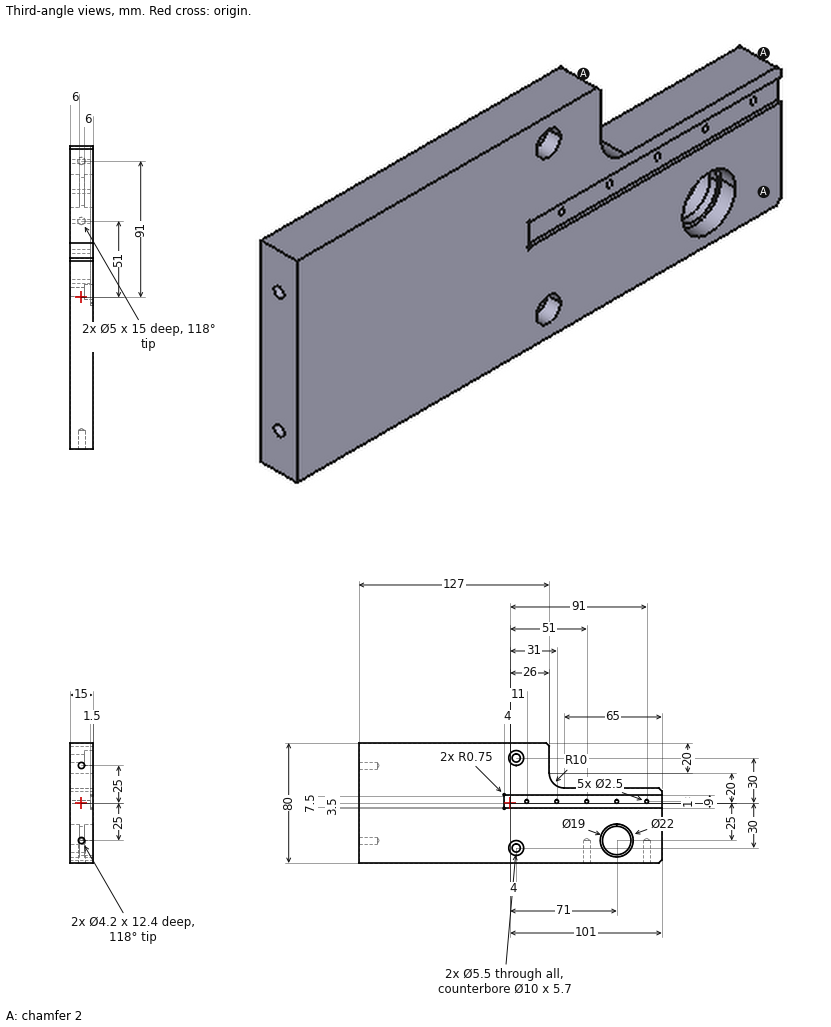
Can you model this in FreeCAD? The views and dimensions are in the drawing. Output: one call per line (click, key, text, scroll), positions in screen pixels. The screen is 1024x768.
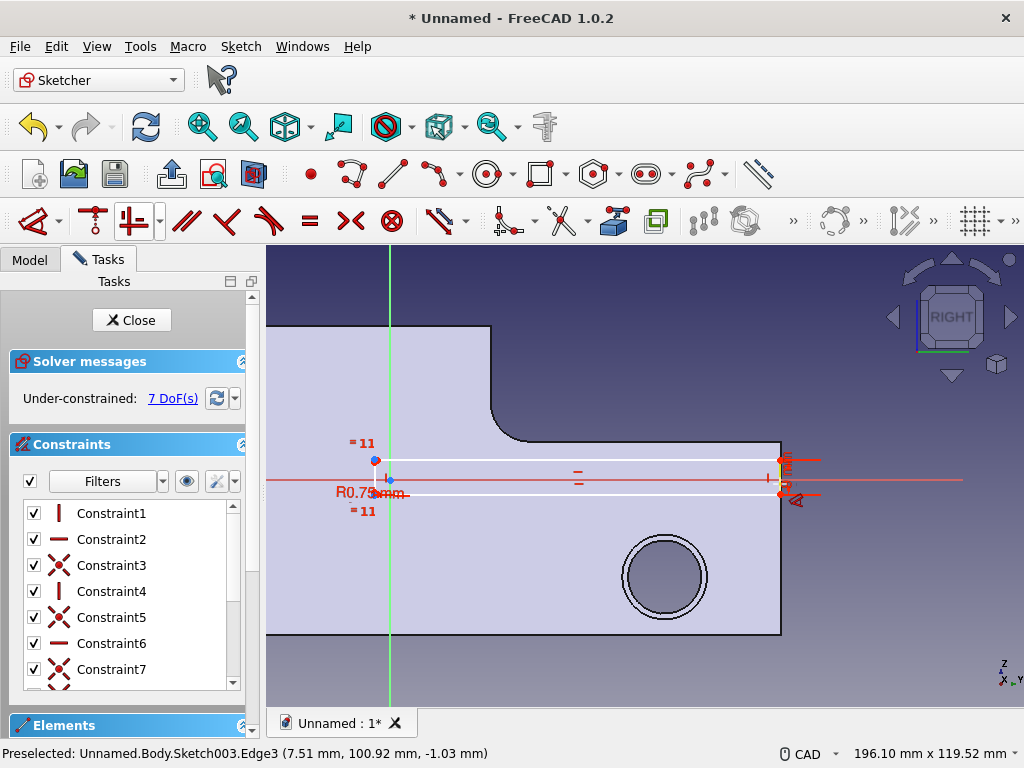
scroll(375, 463, up, 8)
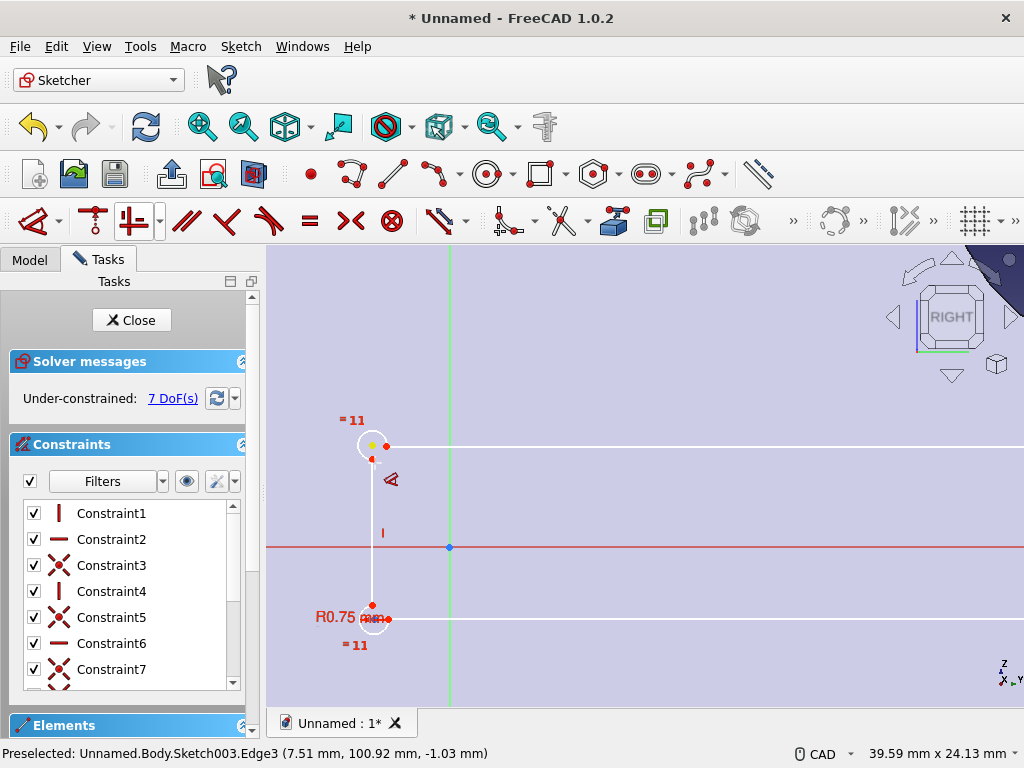
click(372, 459)
click(411, 425)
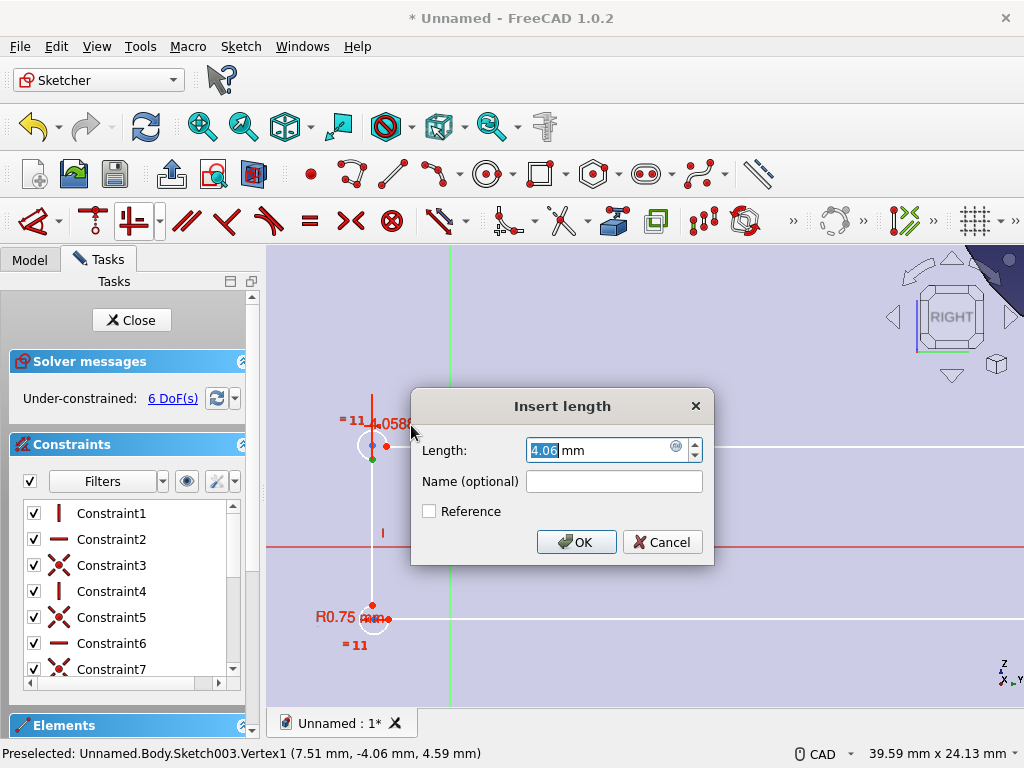
text(4)
key(Return)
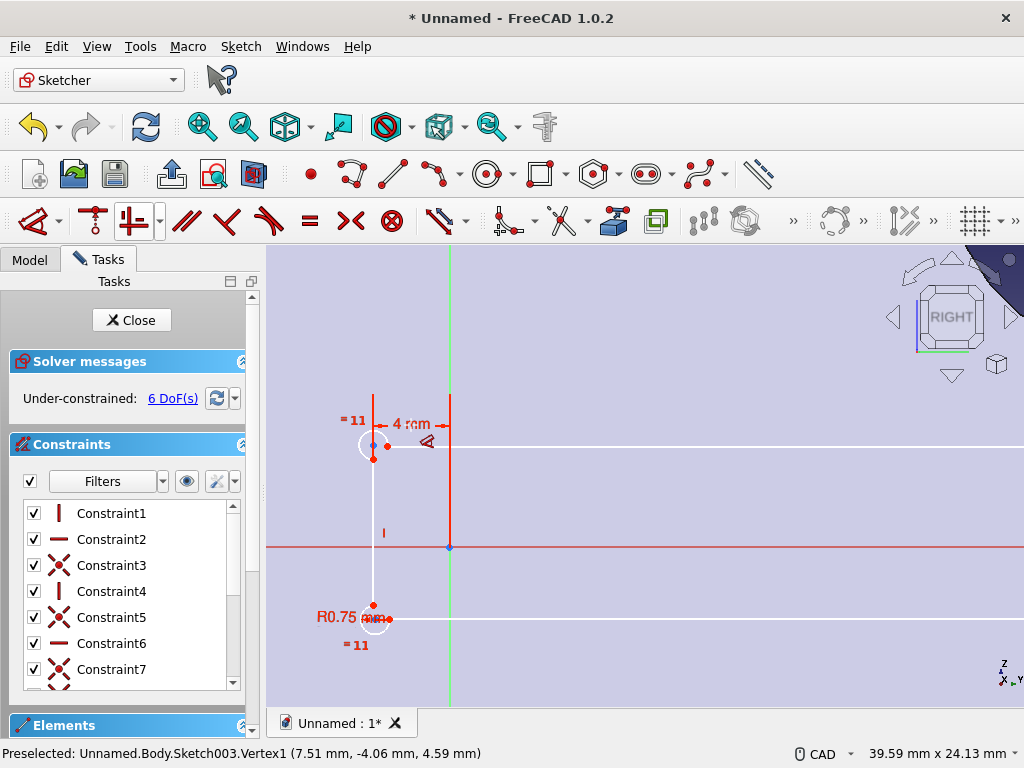
click(375, 620)
click(412, 654)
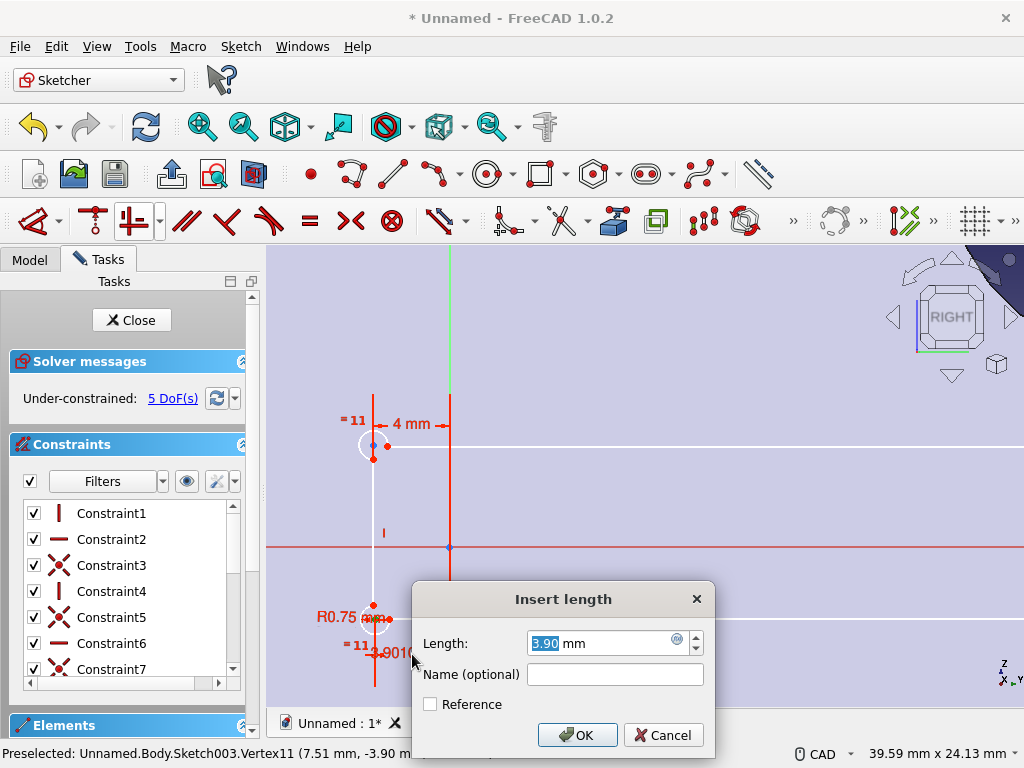
text(4)
key(Return)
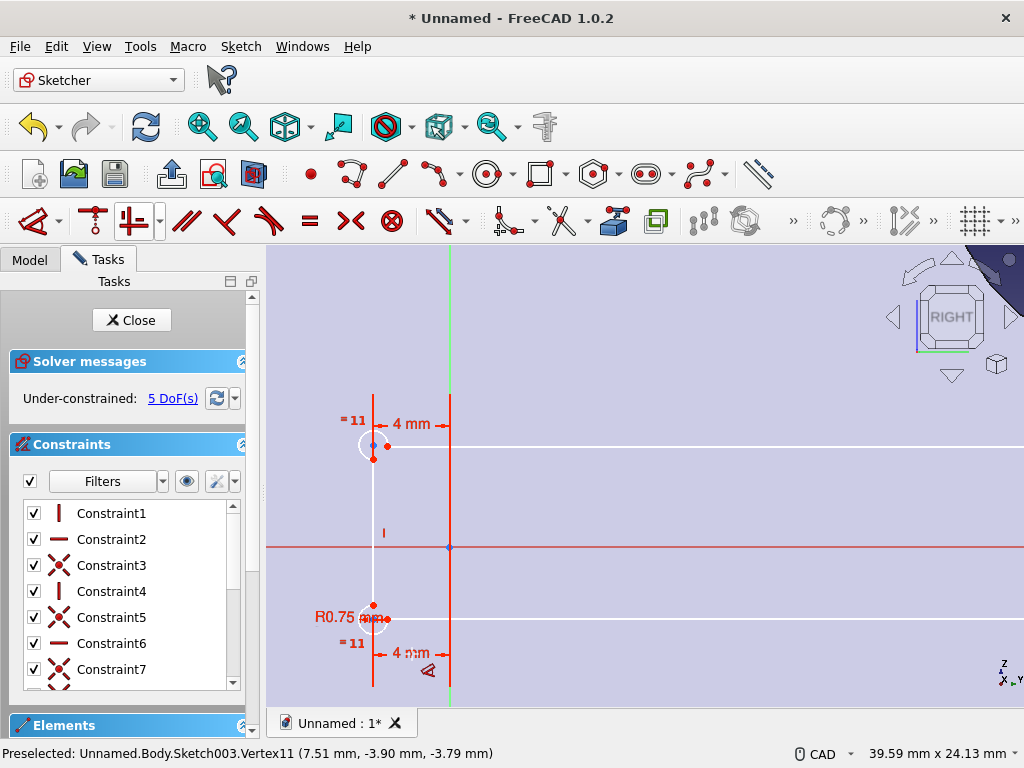
click(374, 445)
click(412, 581)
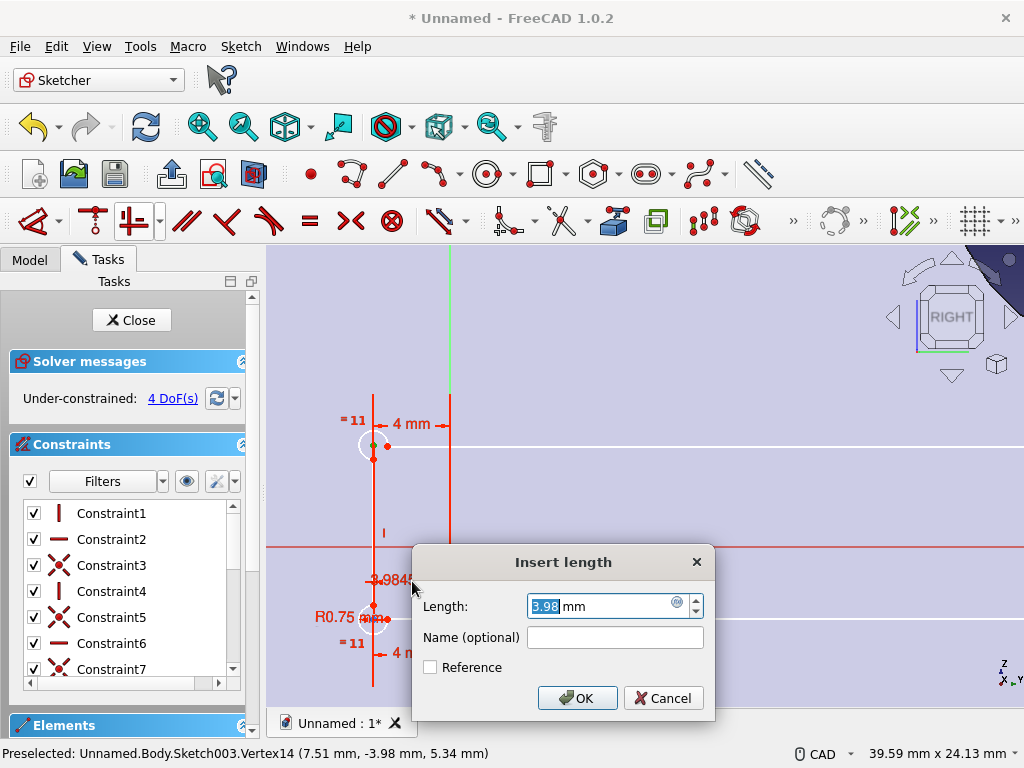
text(4)
key(Return)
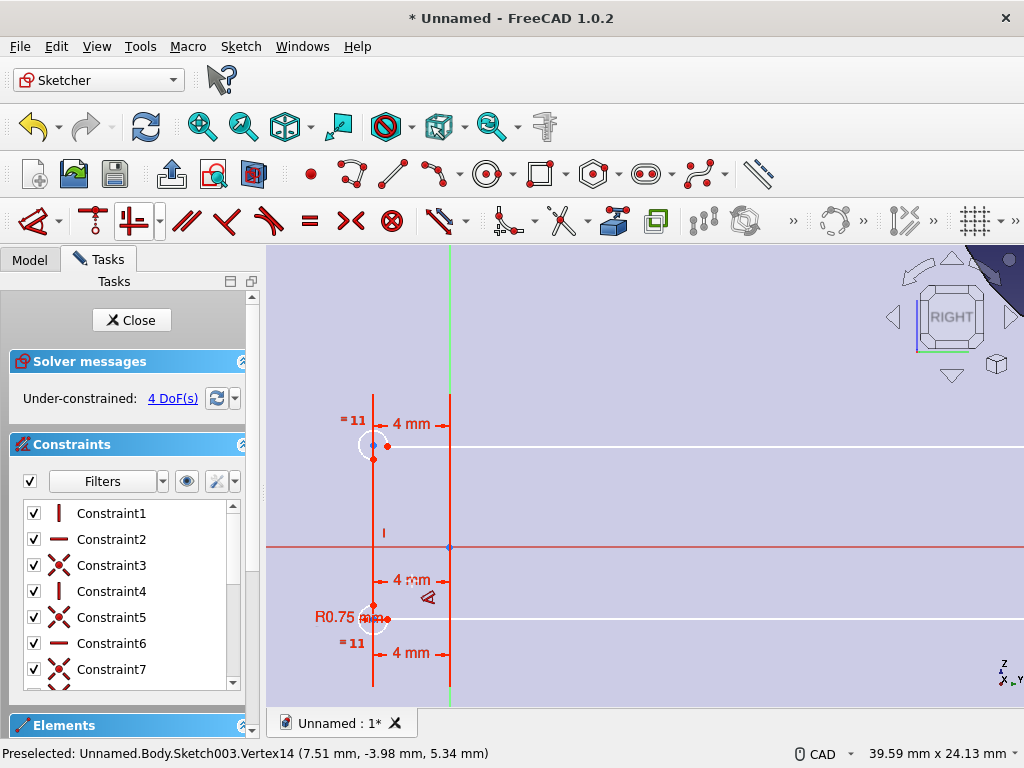
scroll(375, 463, down, 8)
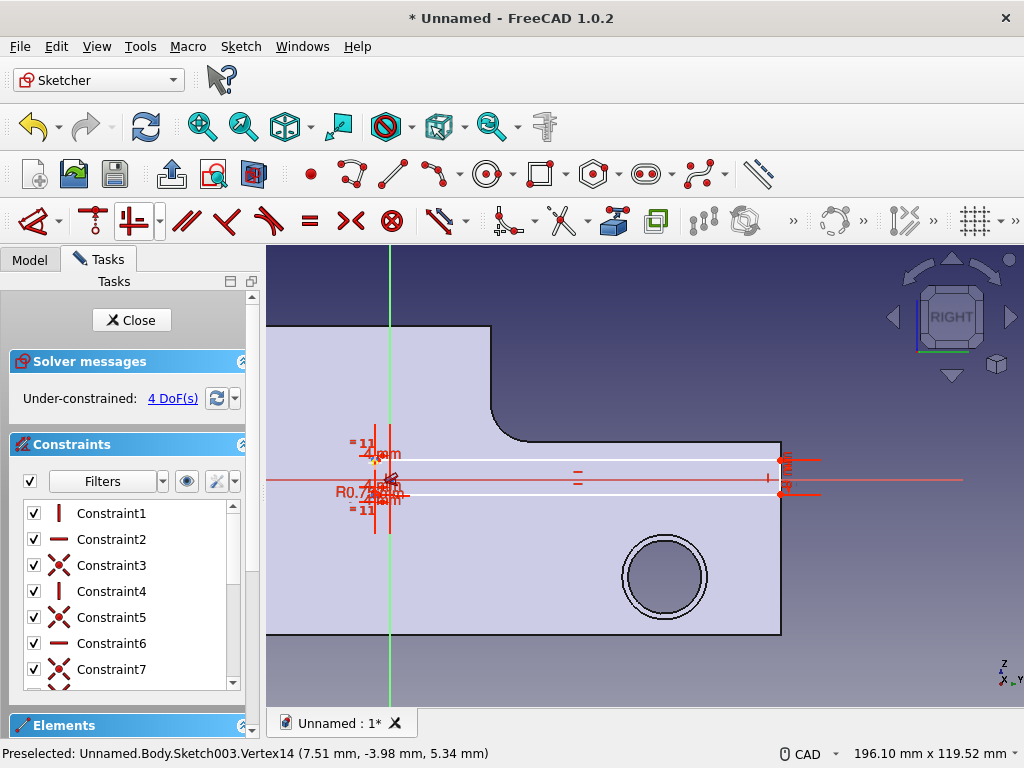
scroll(375, 472, up, 3)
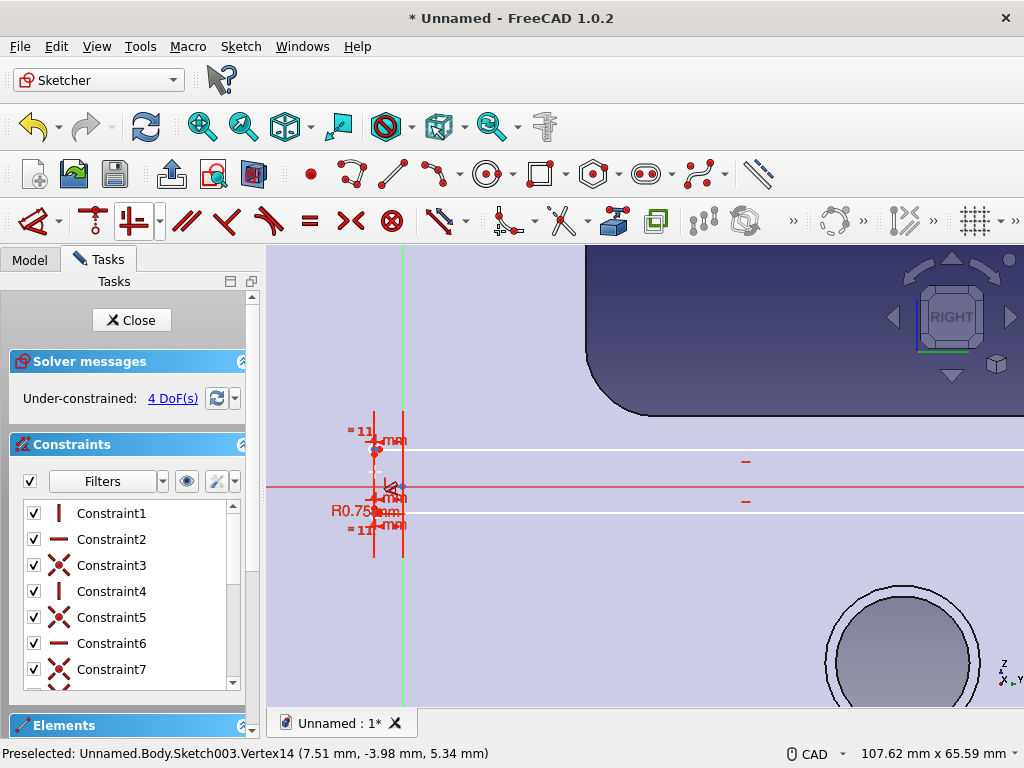
click(374, 471)
click(340, 469)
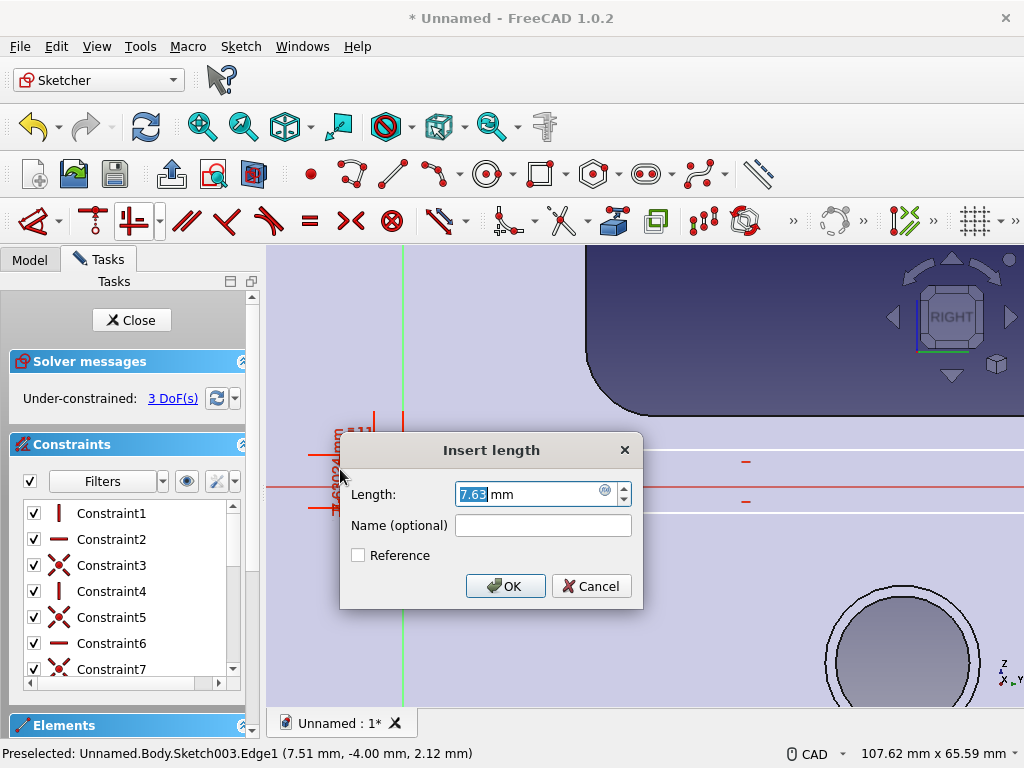
text(7.5)
key(Return)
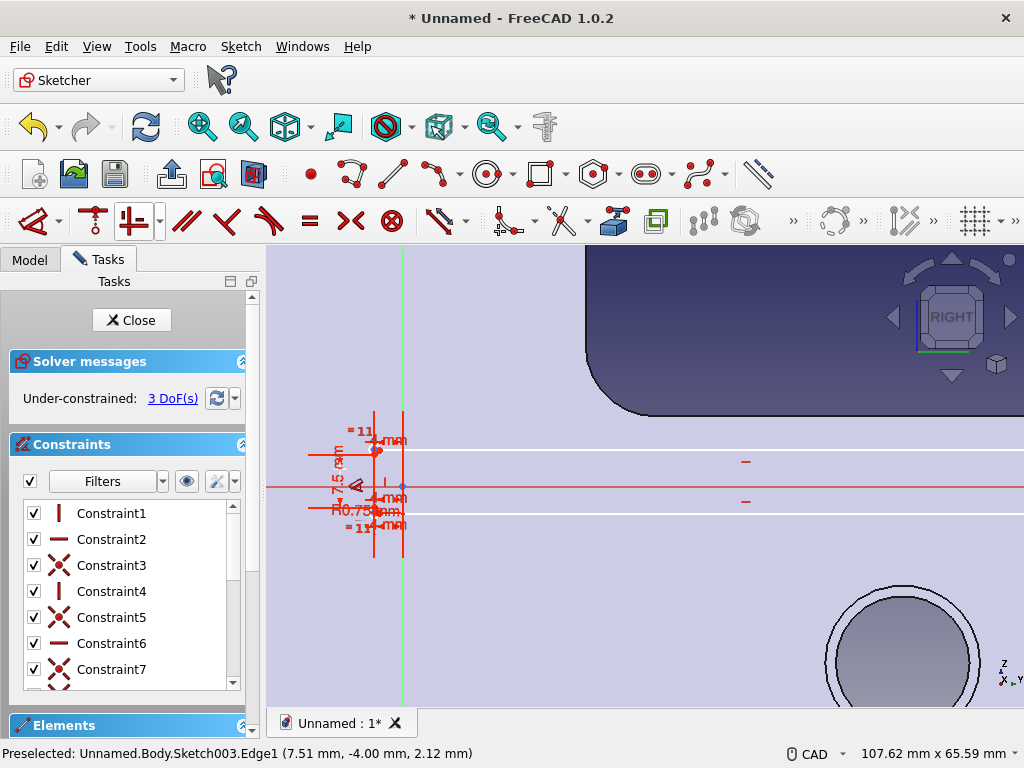
scroll(380, 514, up, 5)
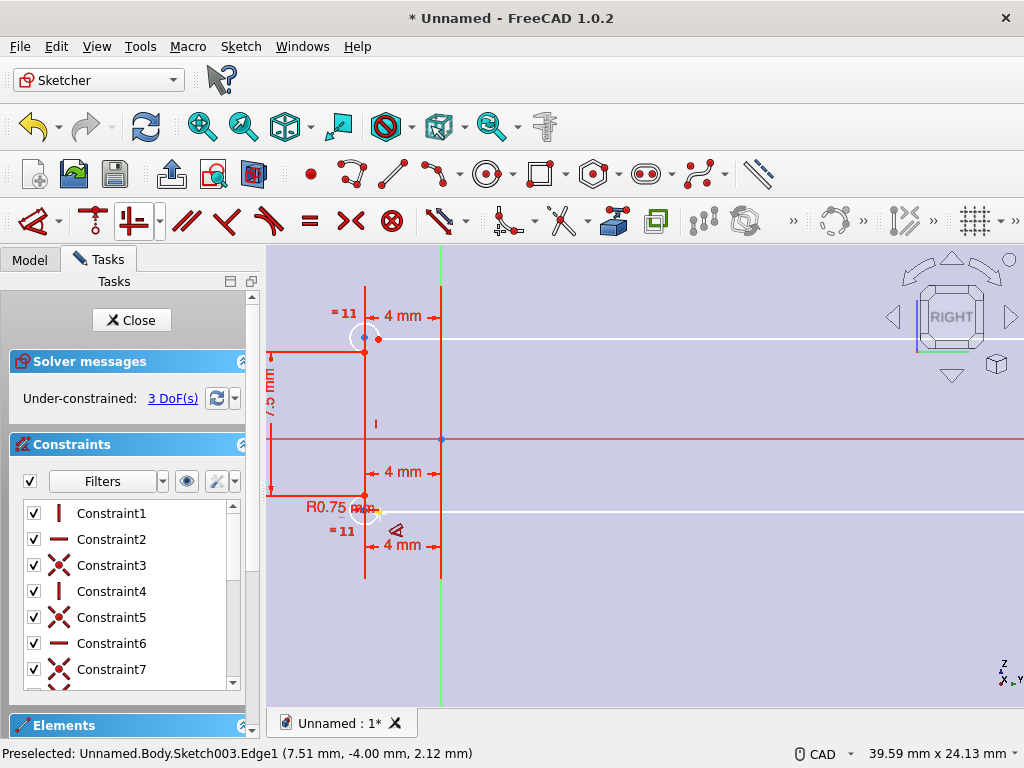
click(379, 512)
click(475, 476)